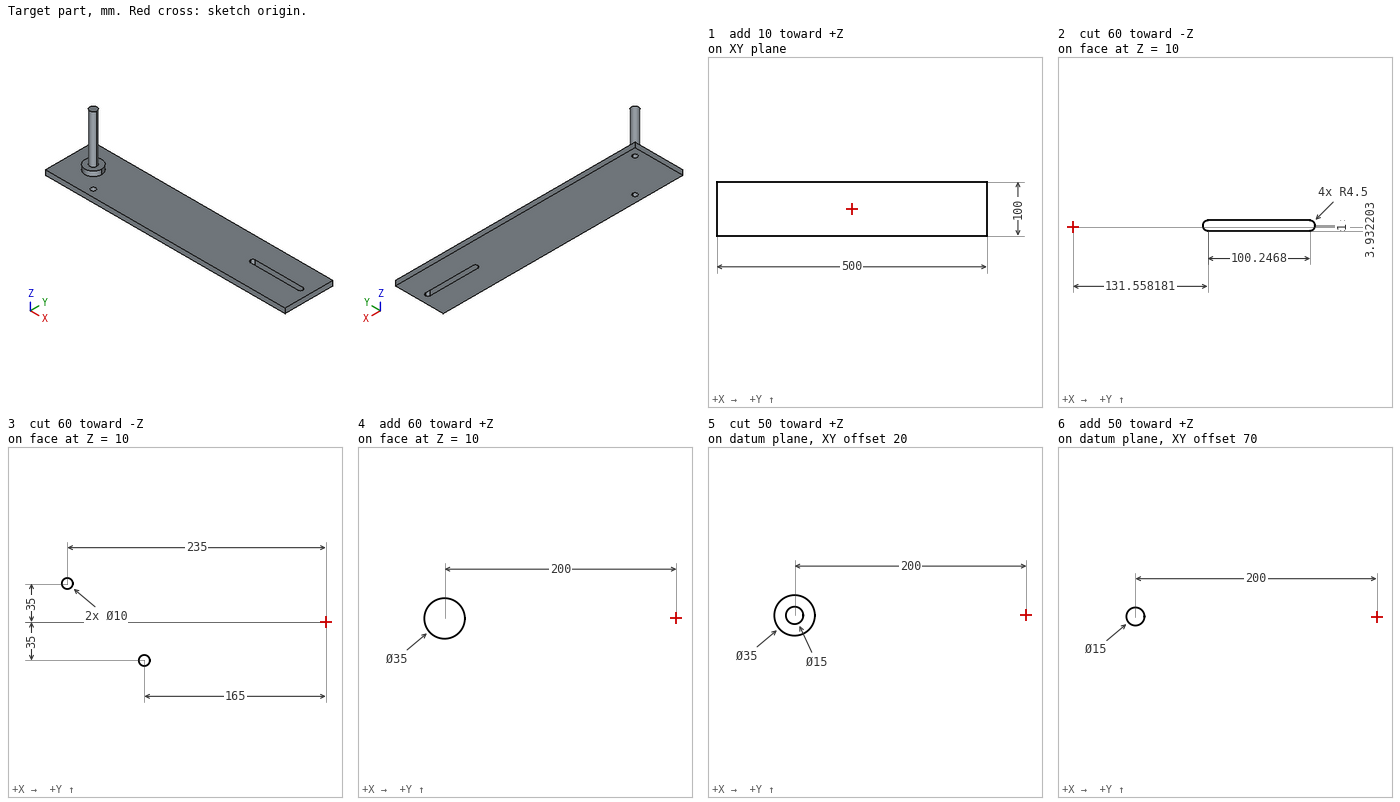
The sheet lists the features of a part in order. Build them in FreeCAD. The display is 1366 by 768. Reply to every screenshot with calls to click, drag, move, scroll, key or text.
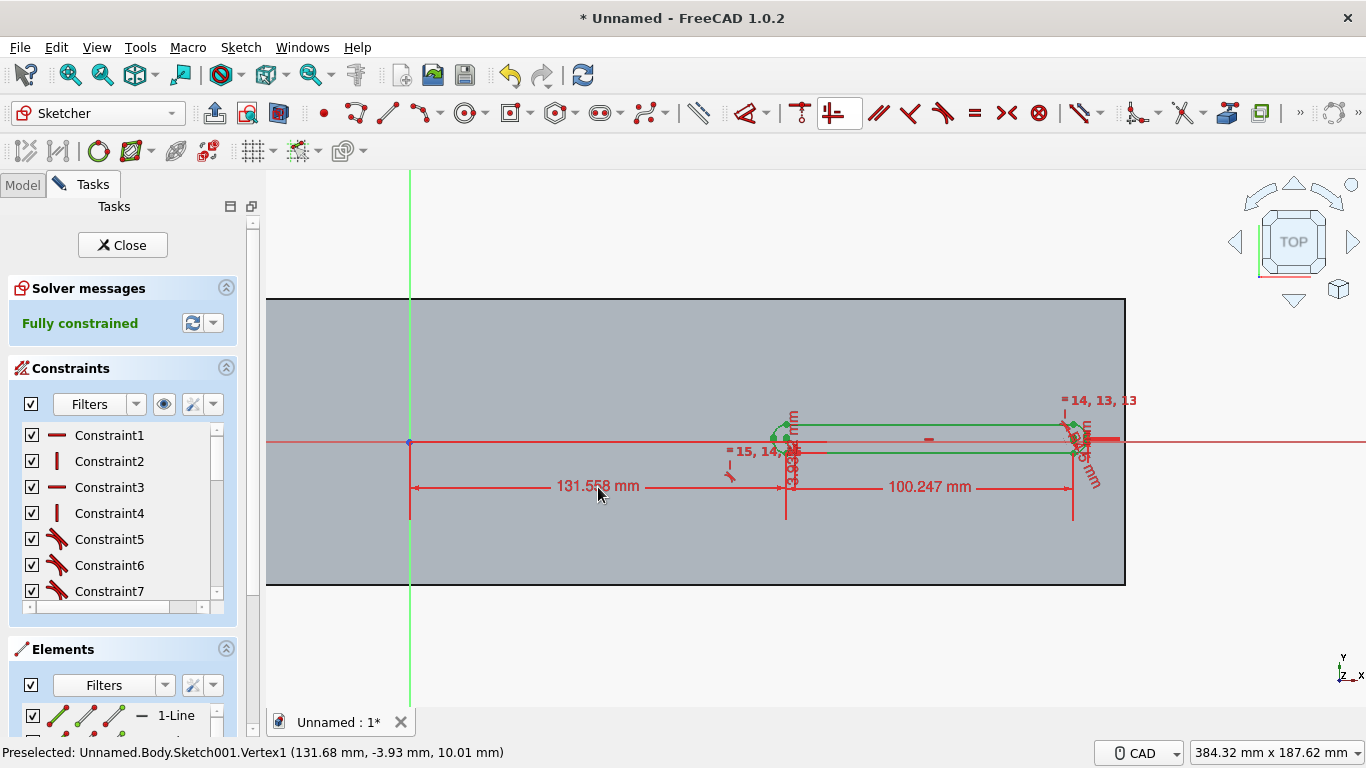
click(123, 245)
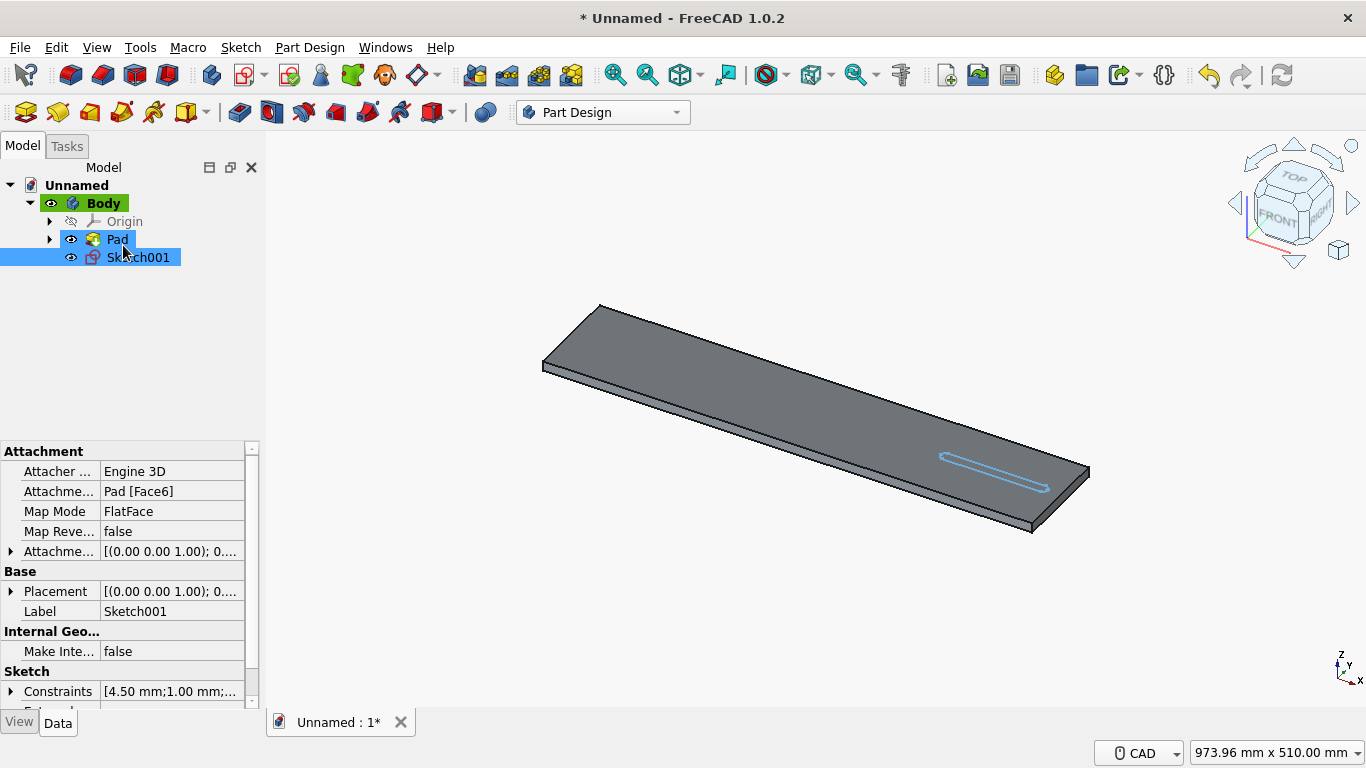
click(240, 112)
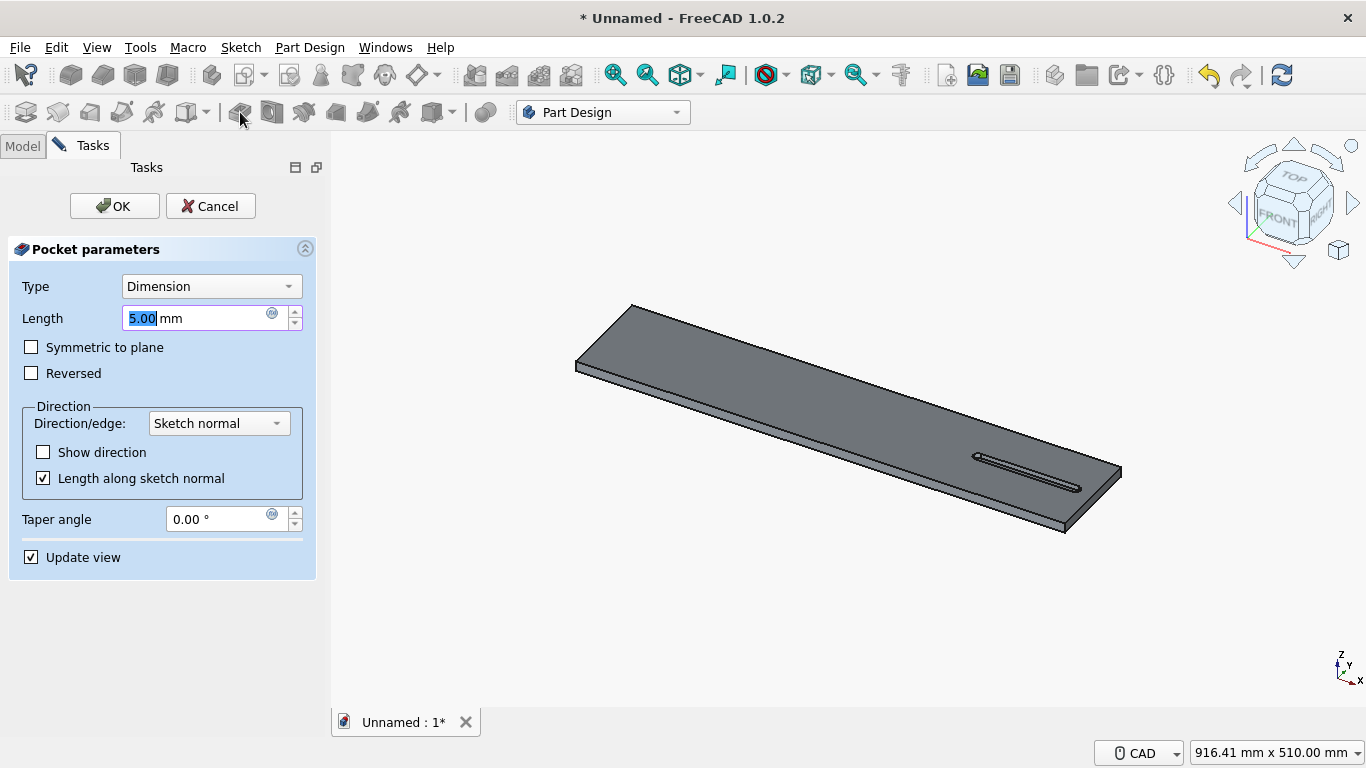
text(60)
key(Tab)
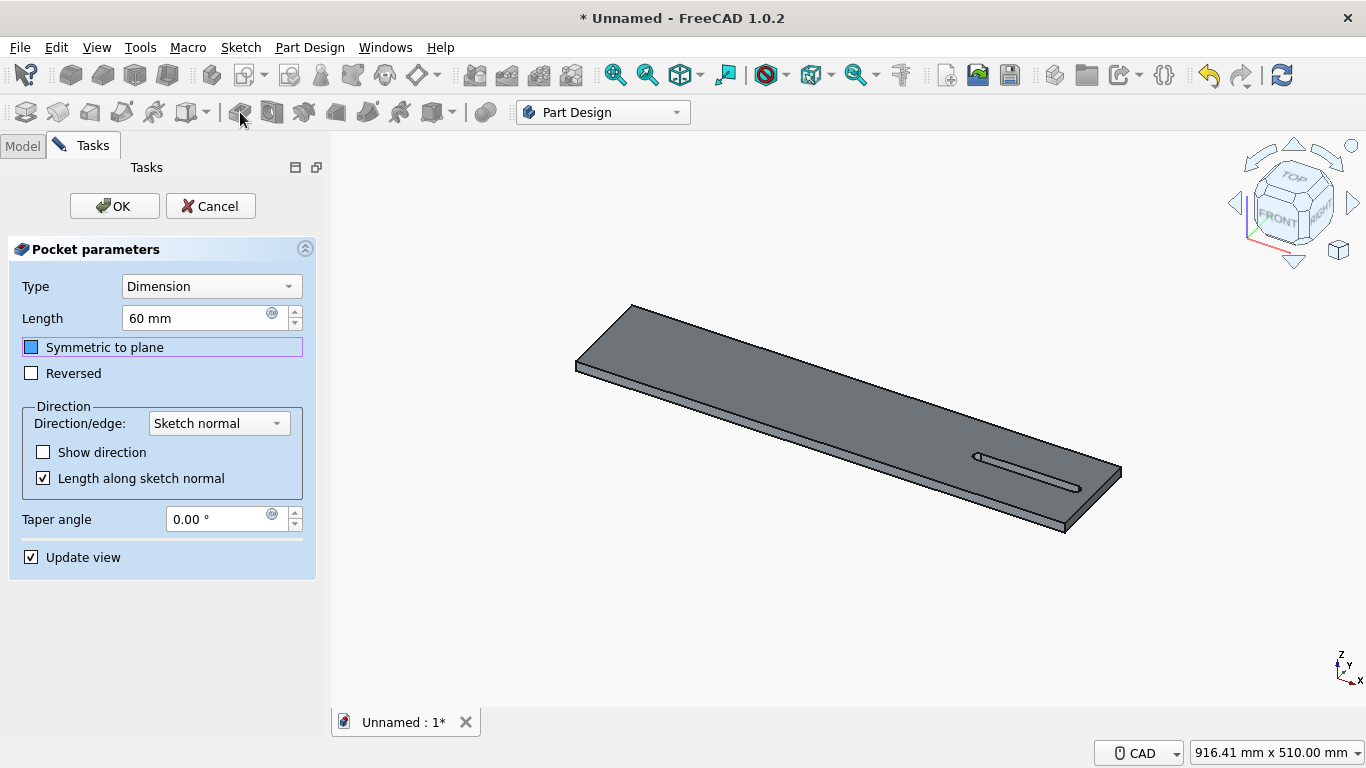
click(115, 206)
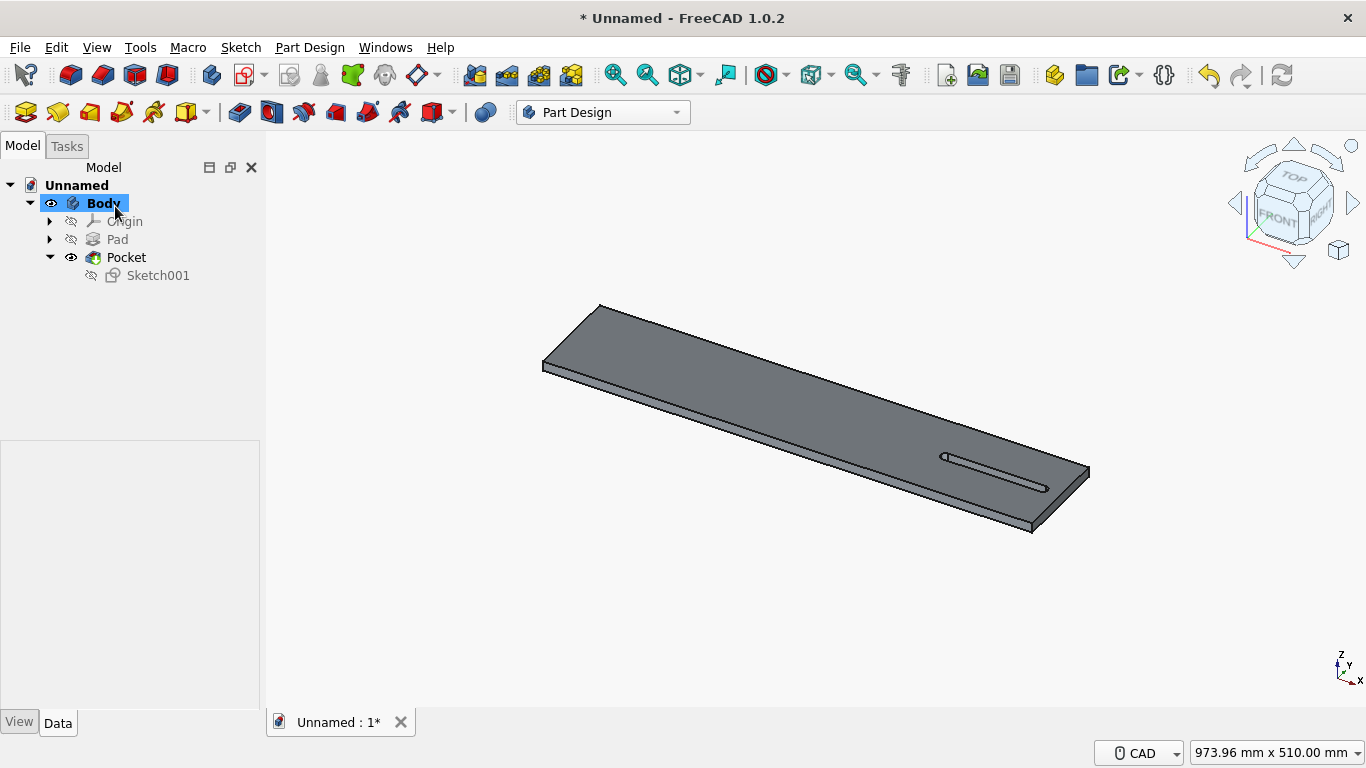
click(886, 437)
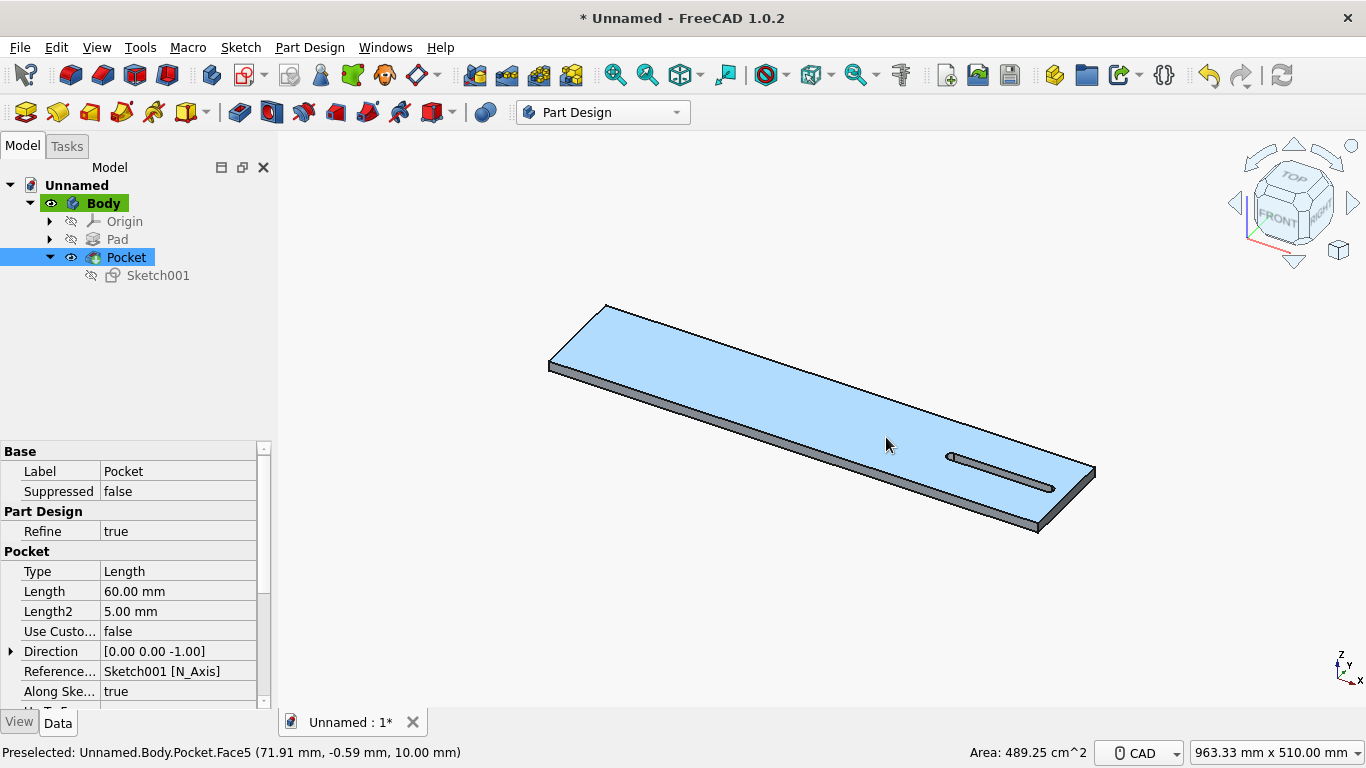
click(244, 76)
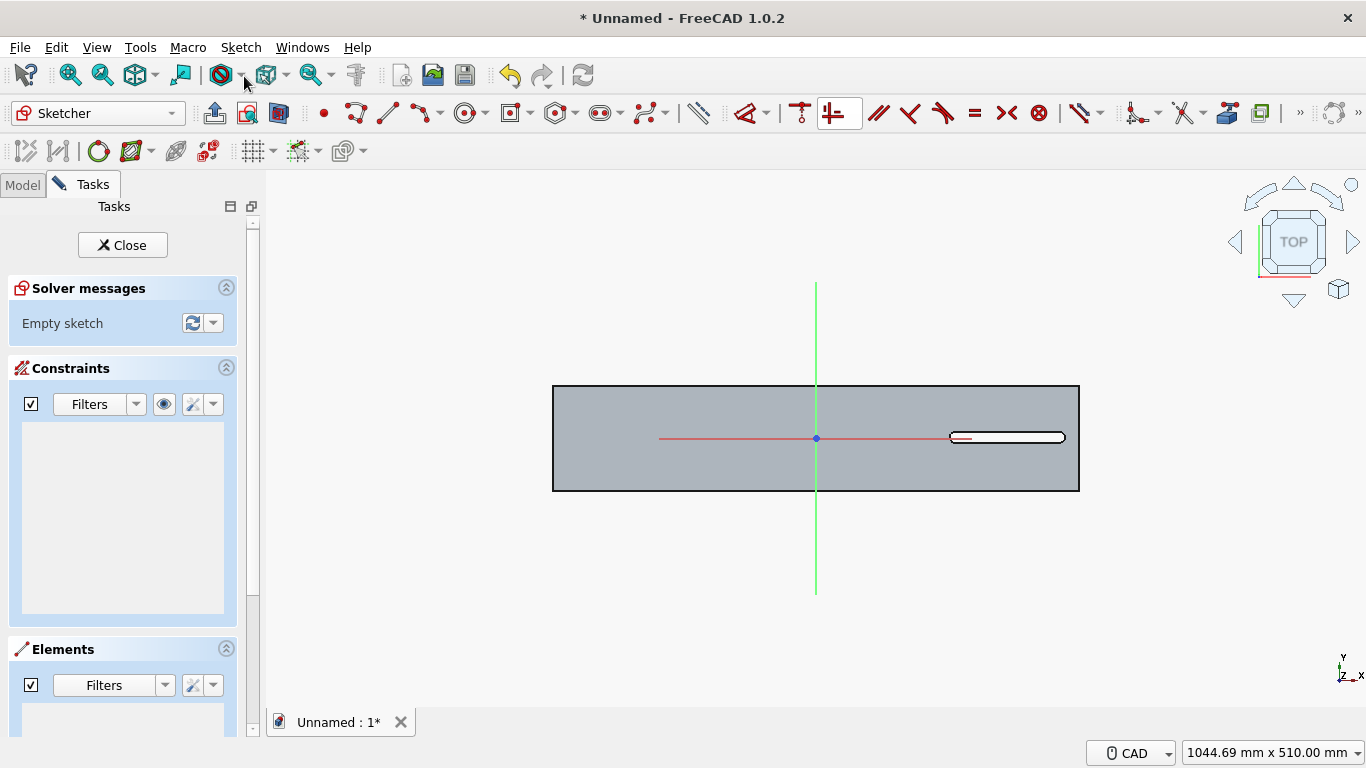
scroll(559, 438, up, 7)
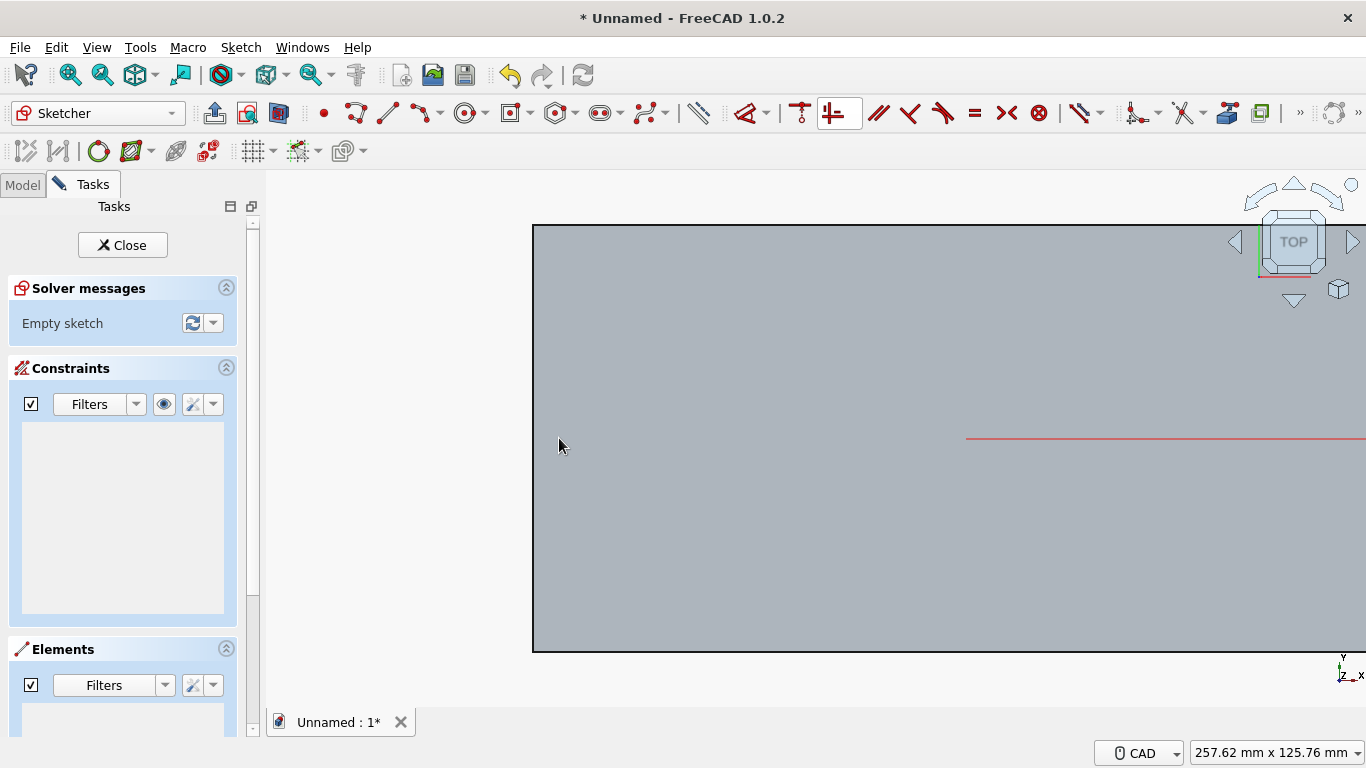
key(g)
key(c)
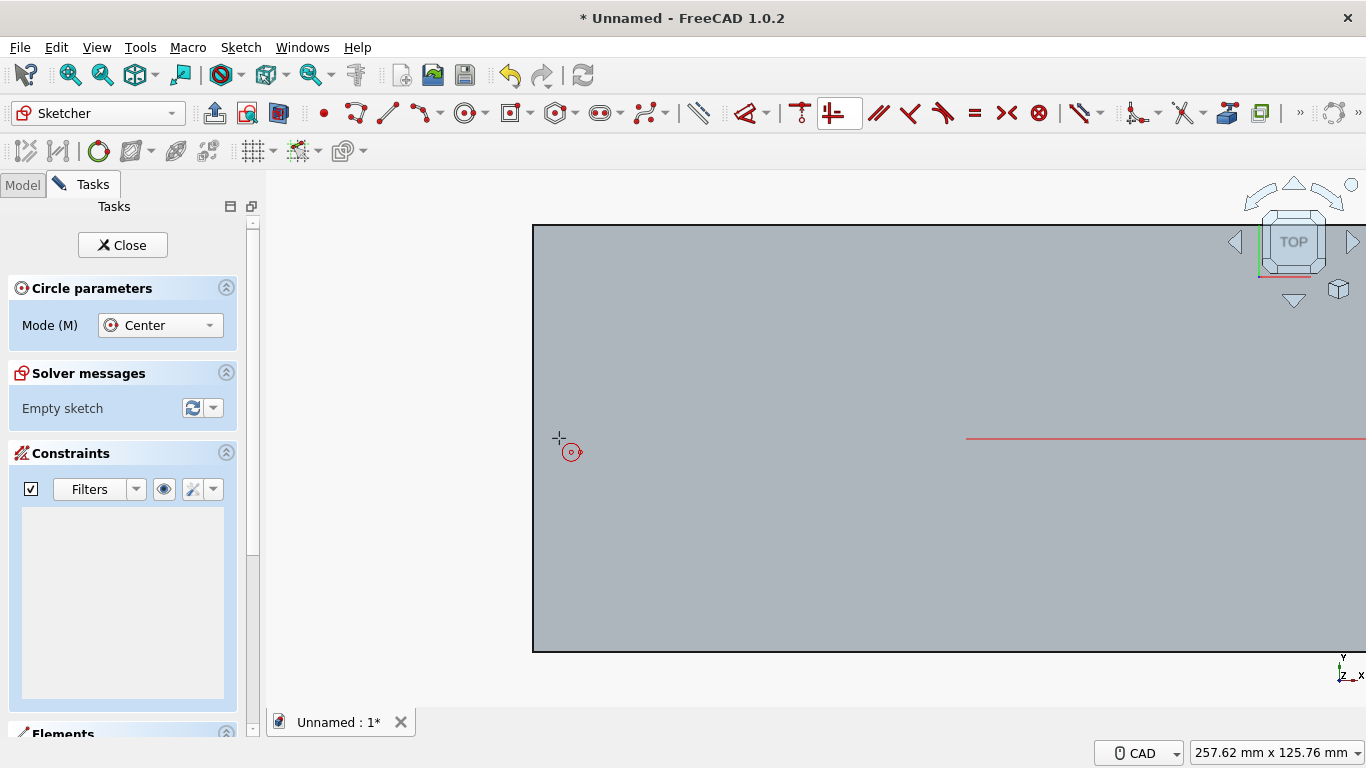
click(597, 289)
move(612, 274)